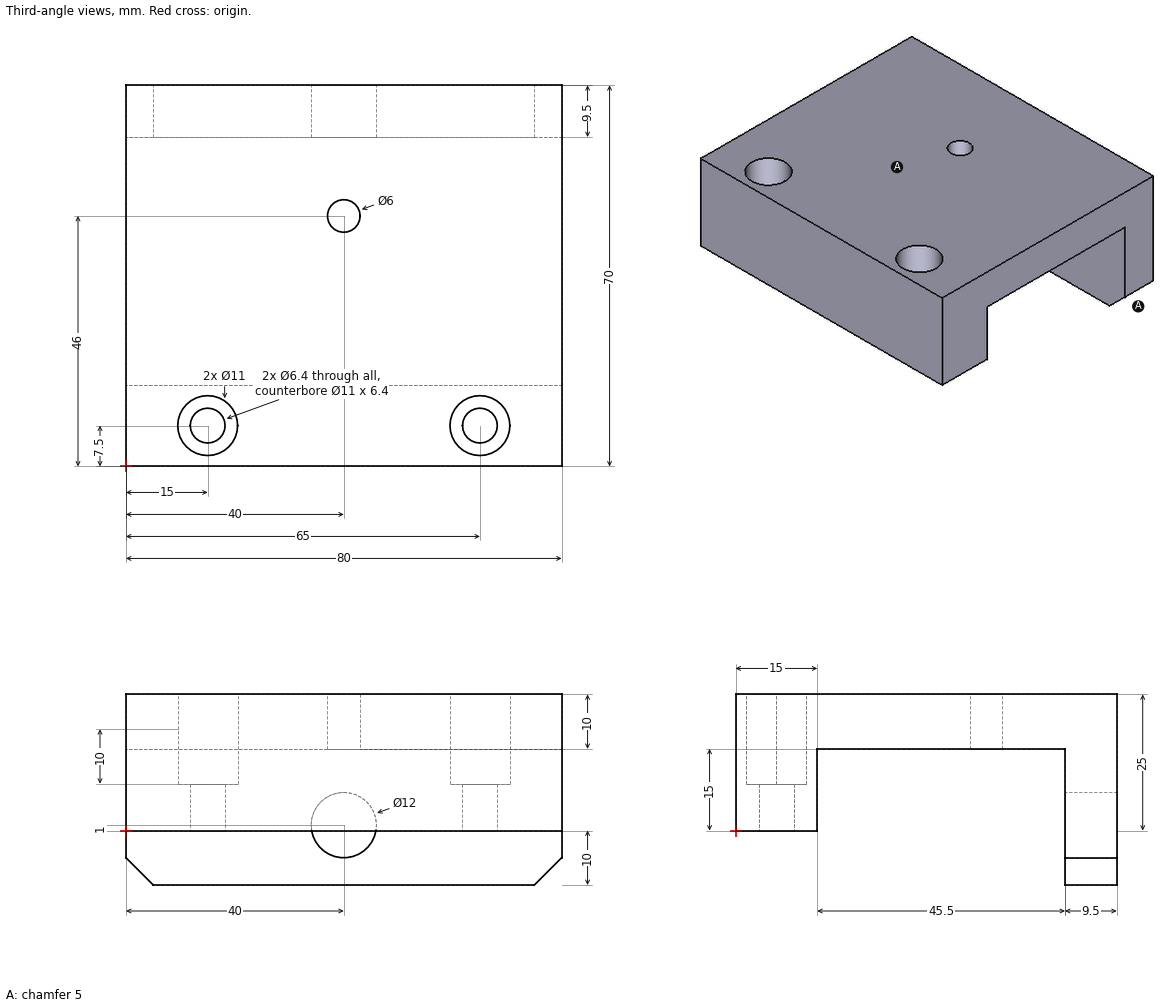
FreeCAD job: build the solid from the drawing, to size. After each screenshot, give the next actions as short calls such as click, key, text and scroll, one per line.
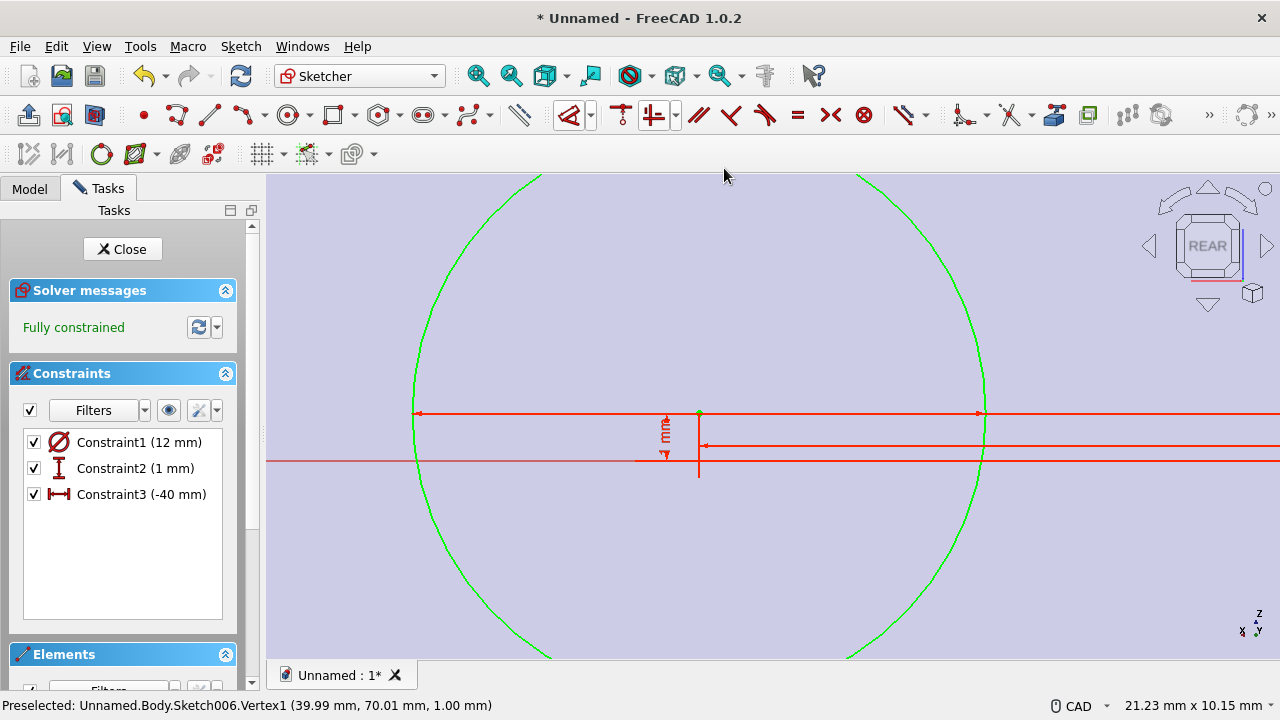
click(123, 249)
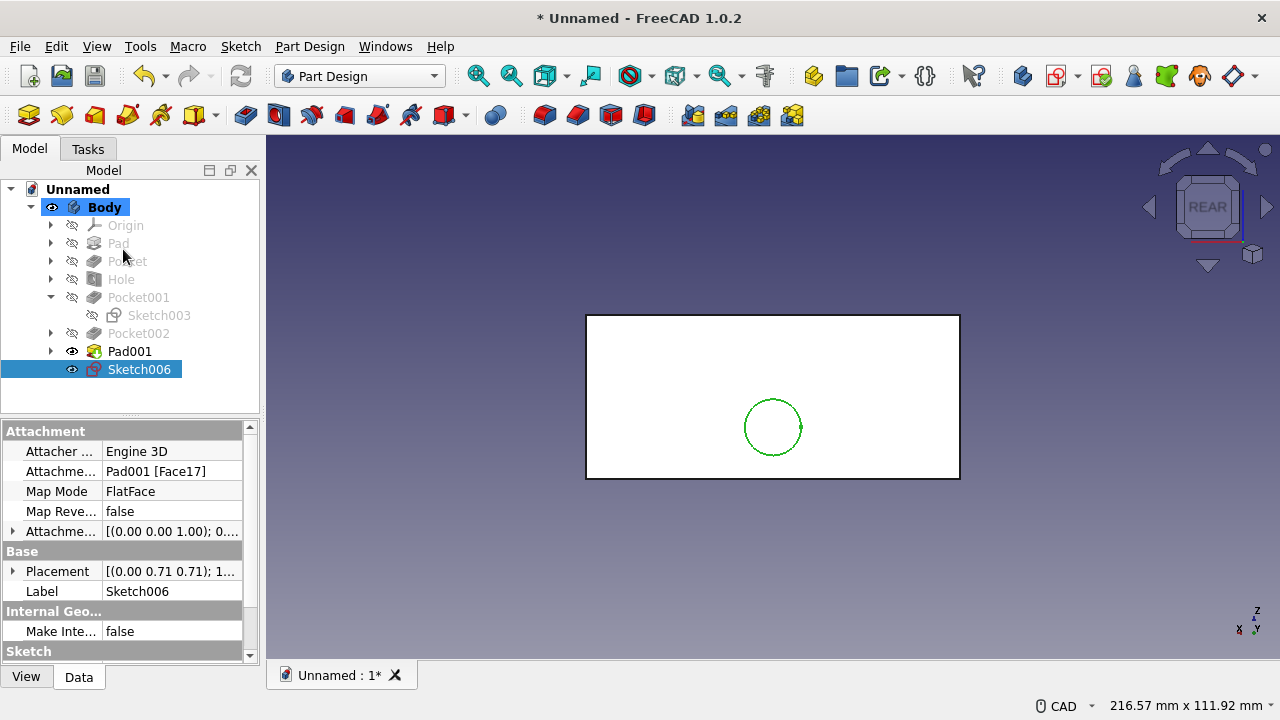
click(246, 116)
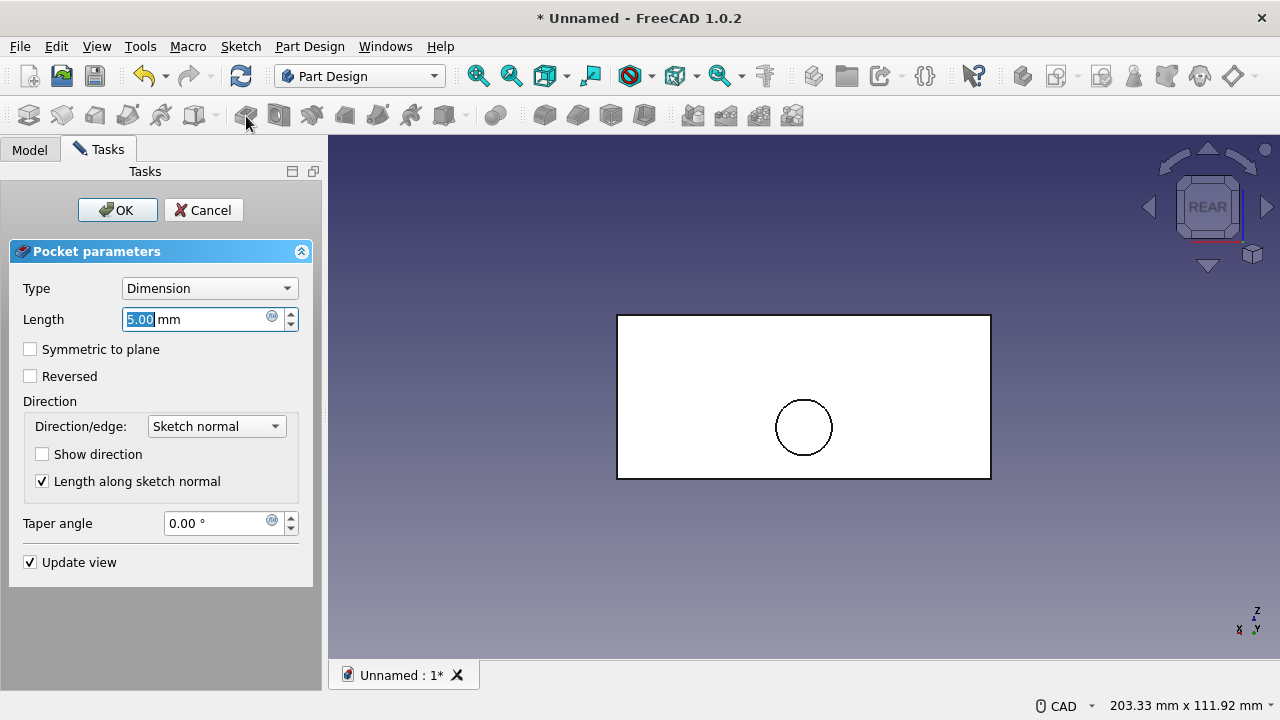
text(9.5)
key(Tab)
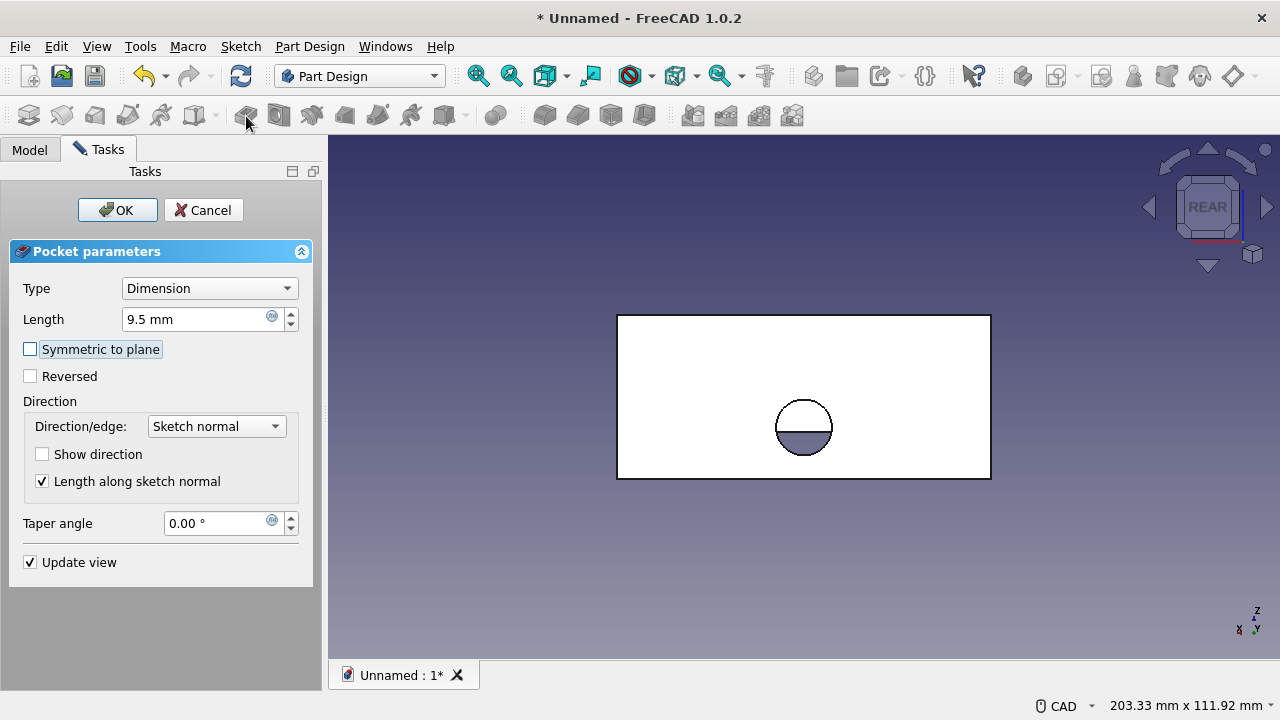
click(118, 210)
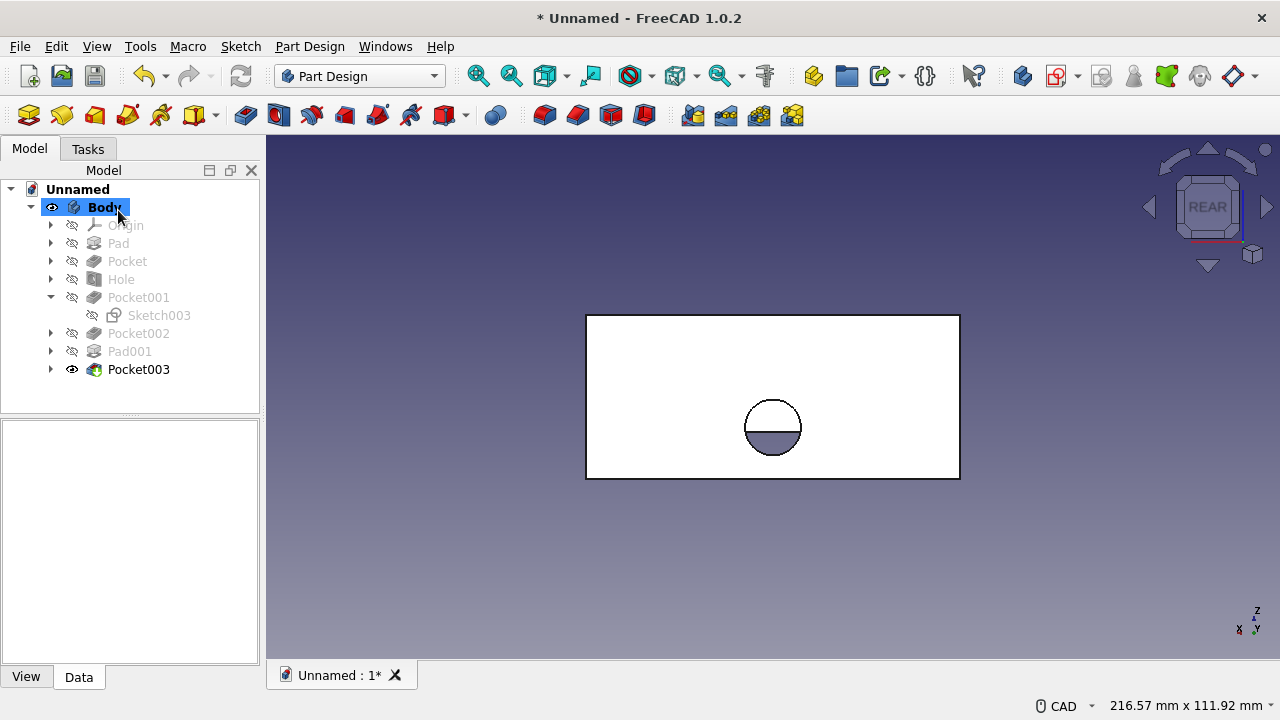
click(479, 76)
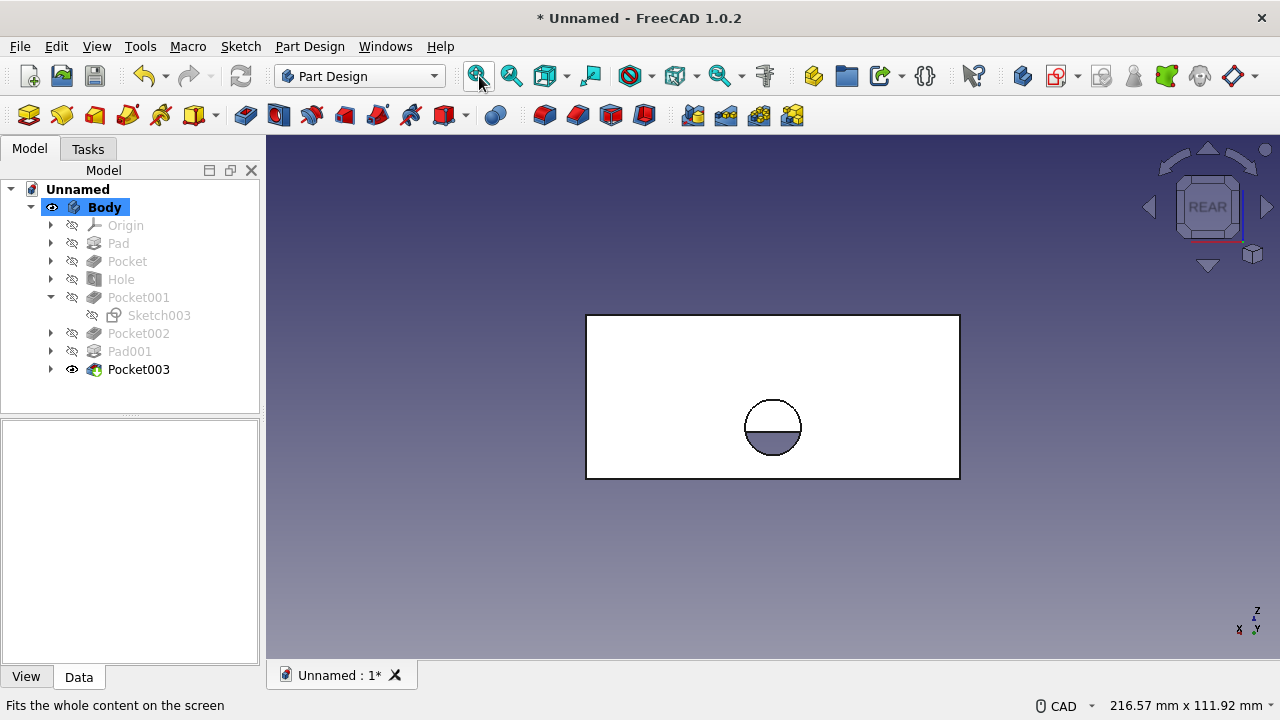
key(0)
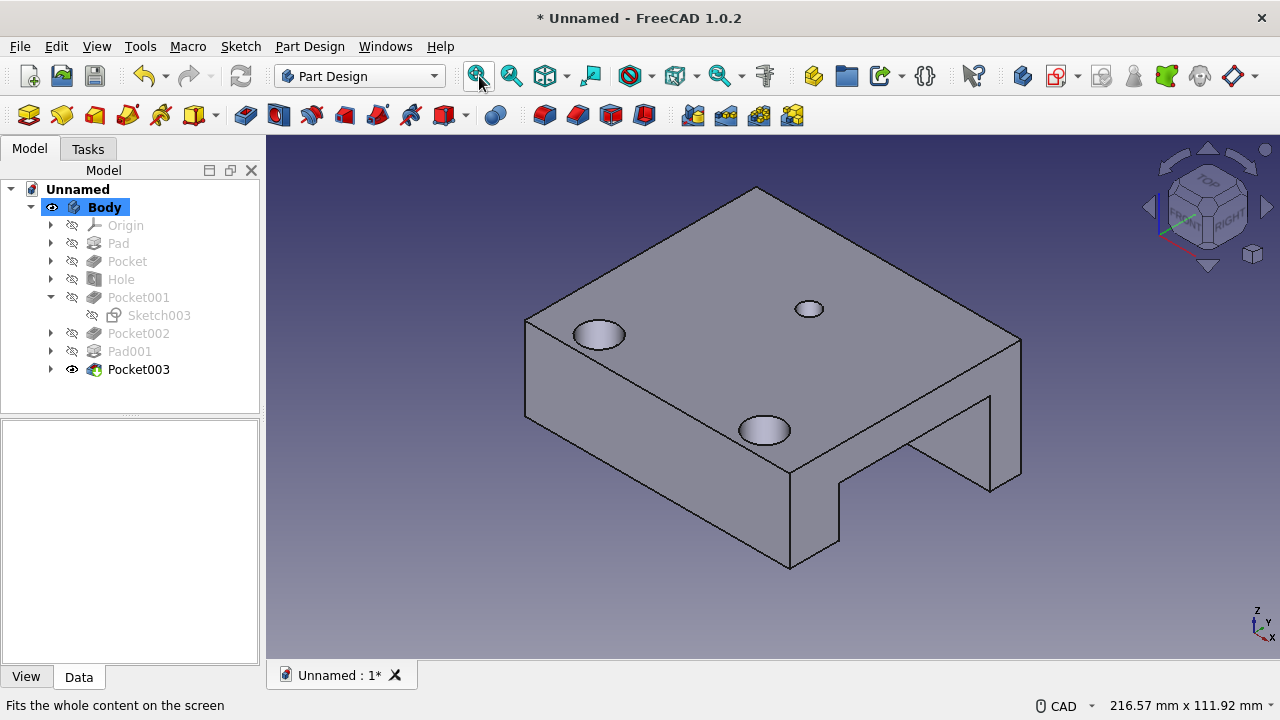
key(2)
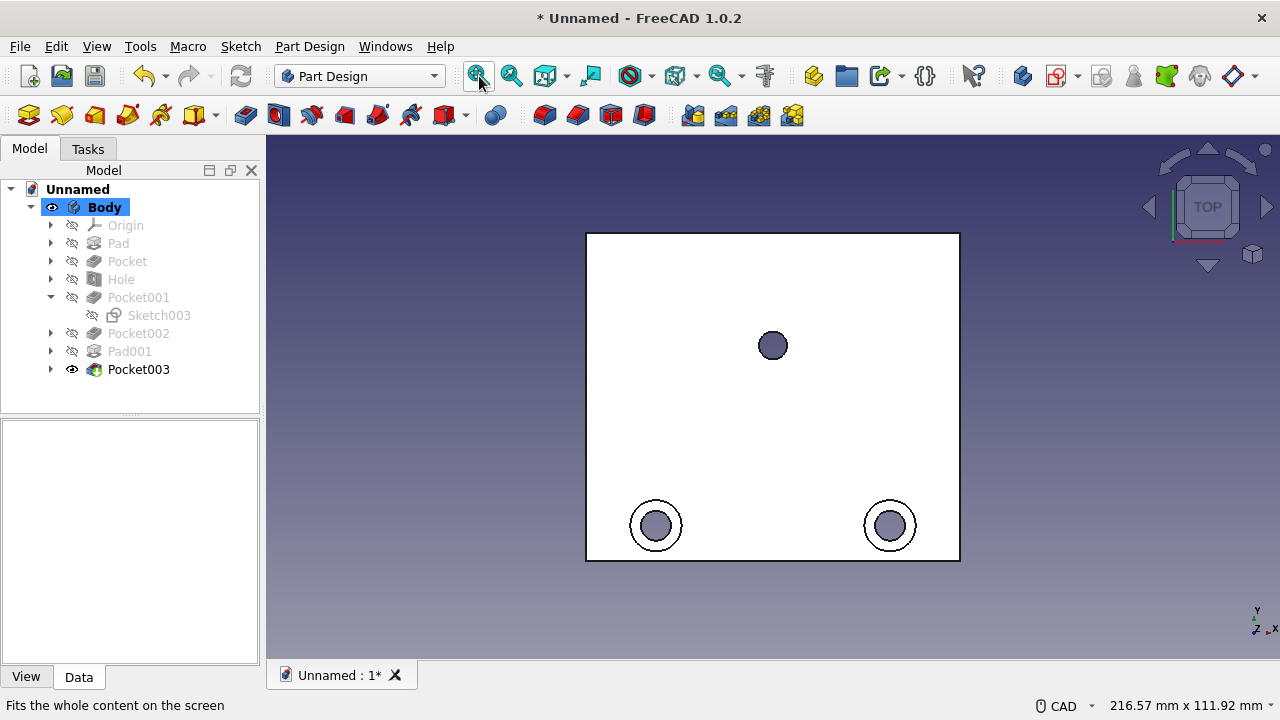
key(1)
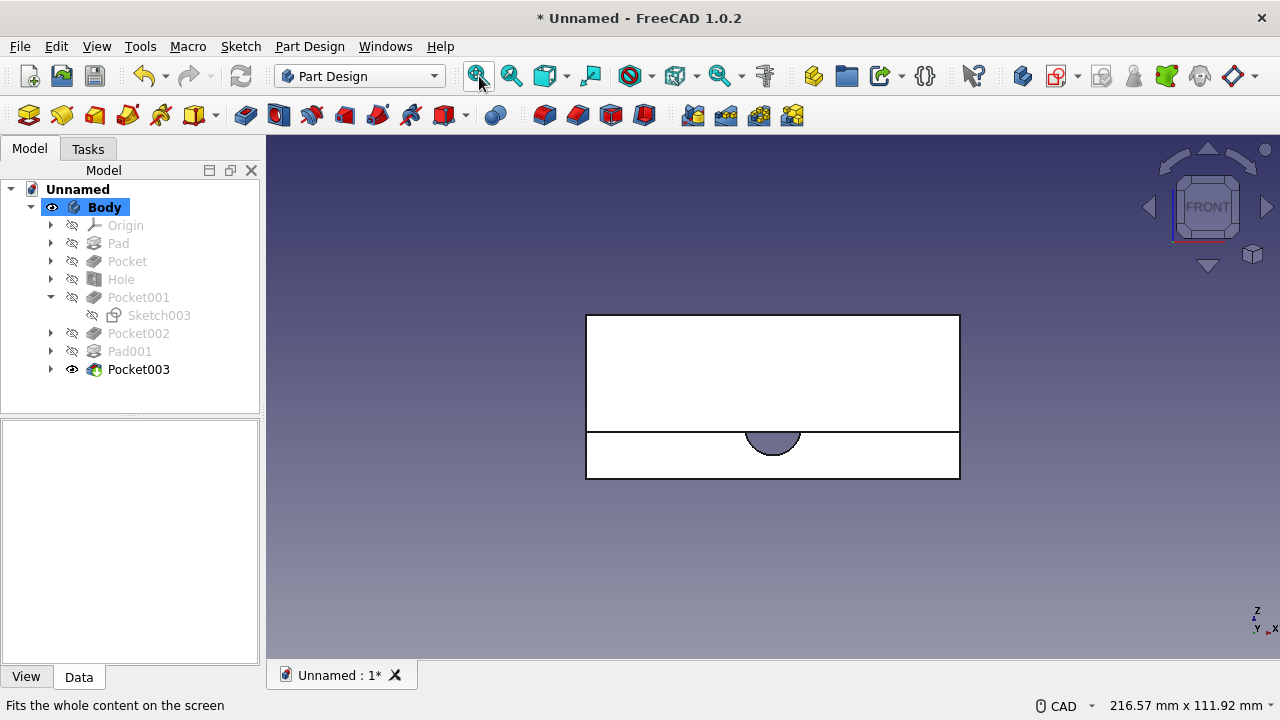
click(479, 76)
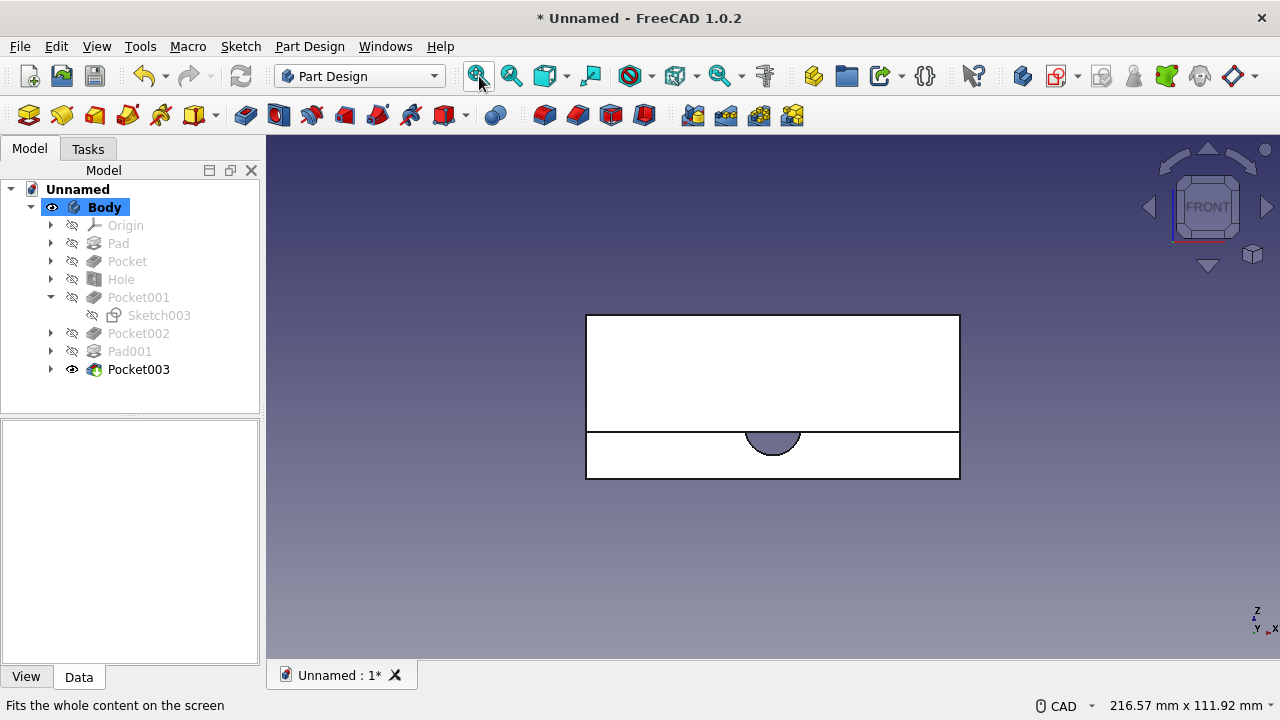
key(3)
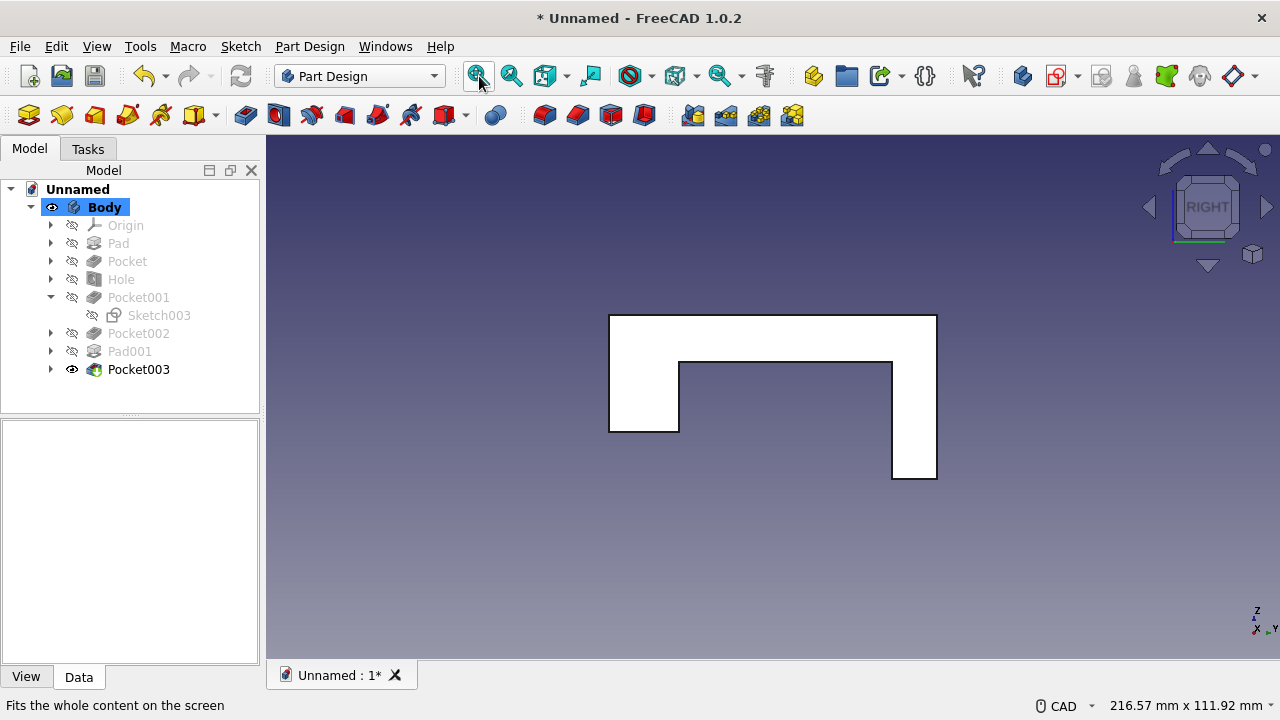
click(479, 76)